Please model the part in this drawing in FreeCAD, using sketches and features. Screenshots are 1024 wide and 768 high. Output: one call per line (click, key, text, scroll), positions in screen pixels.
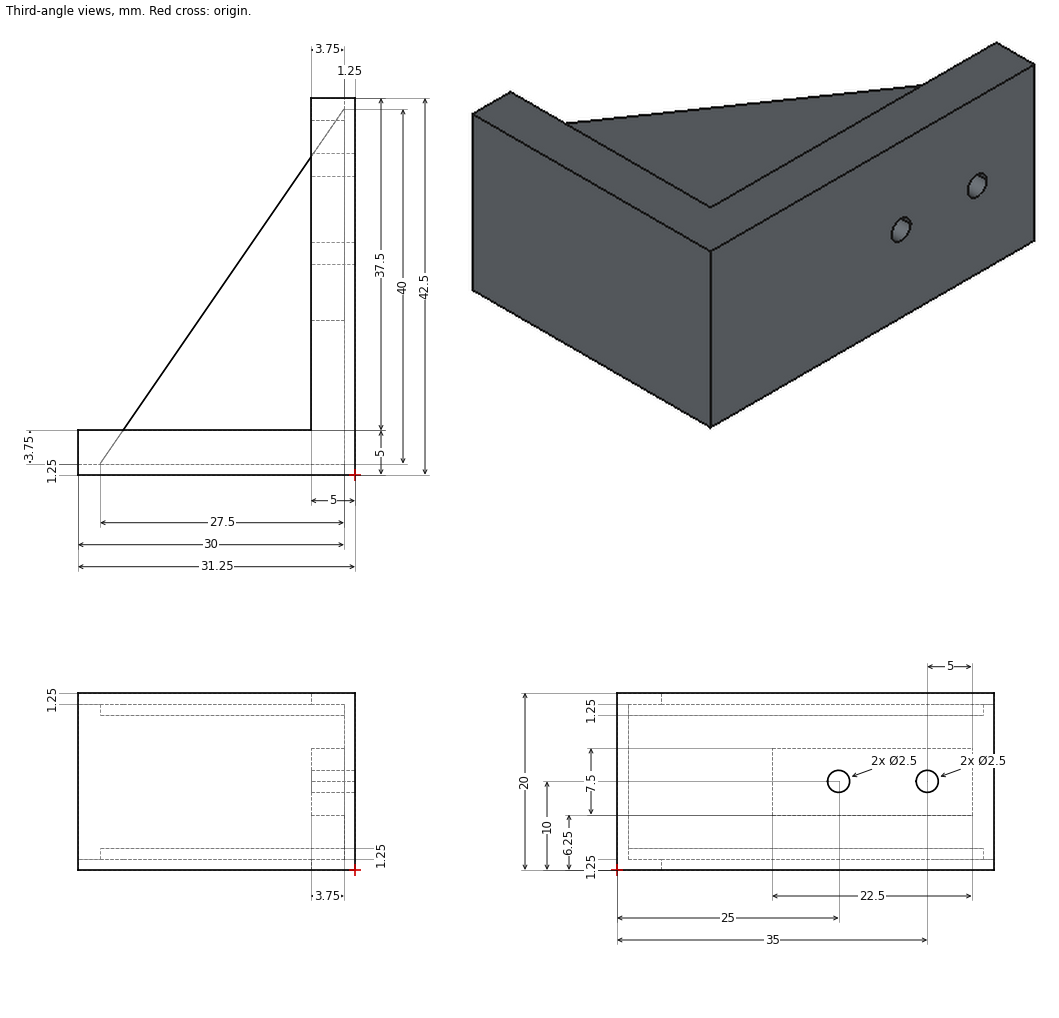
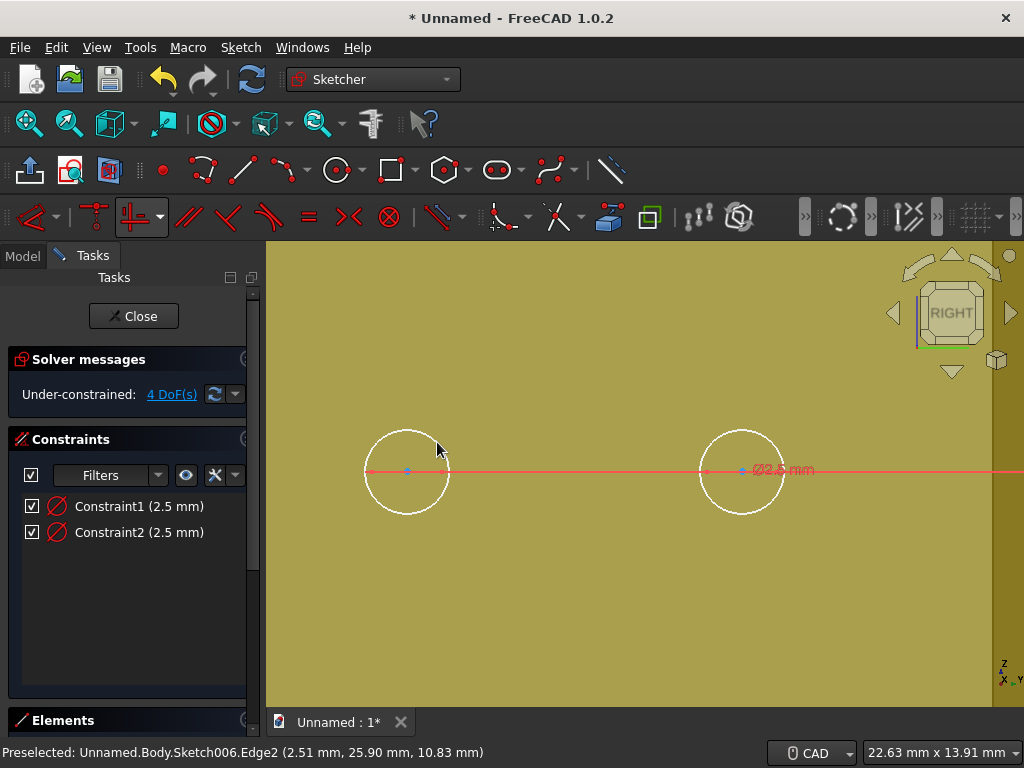
click(742, 472)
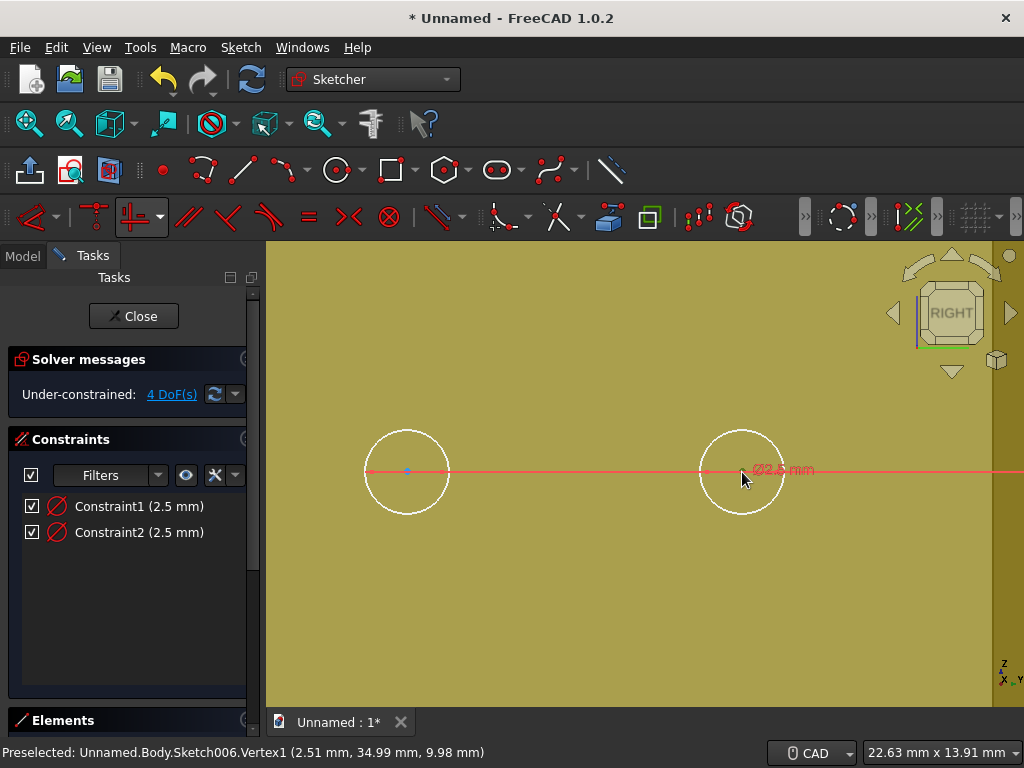
click(407, 472)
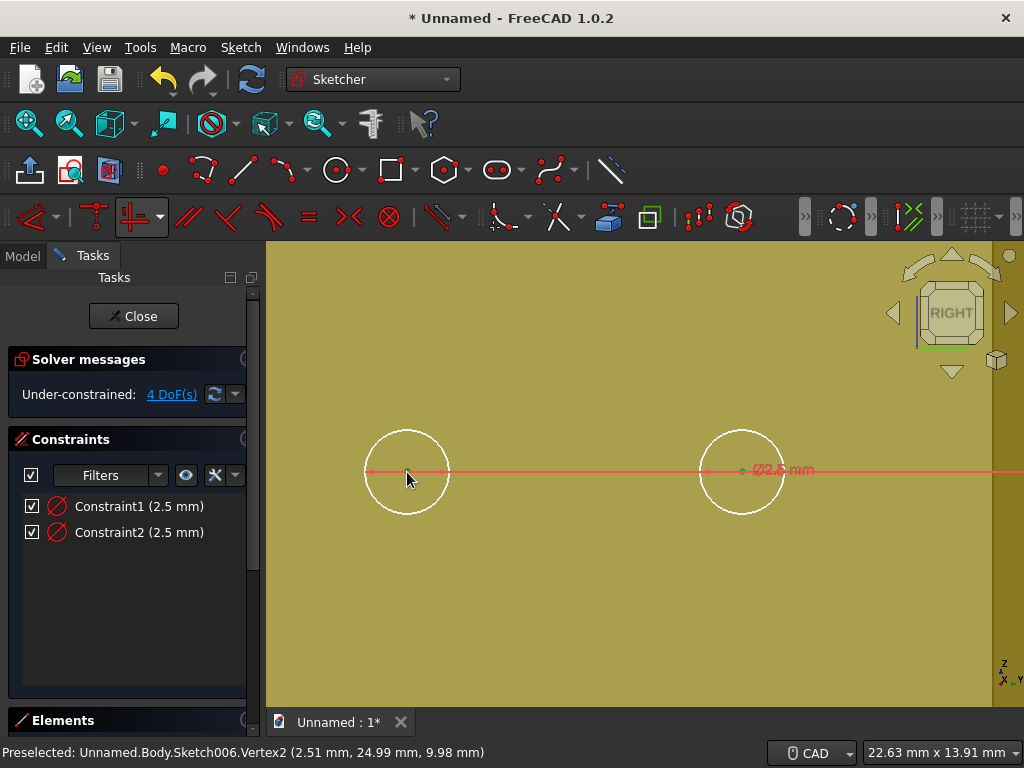
click(162, 218)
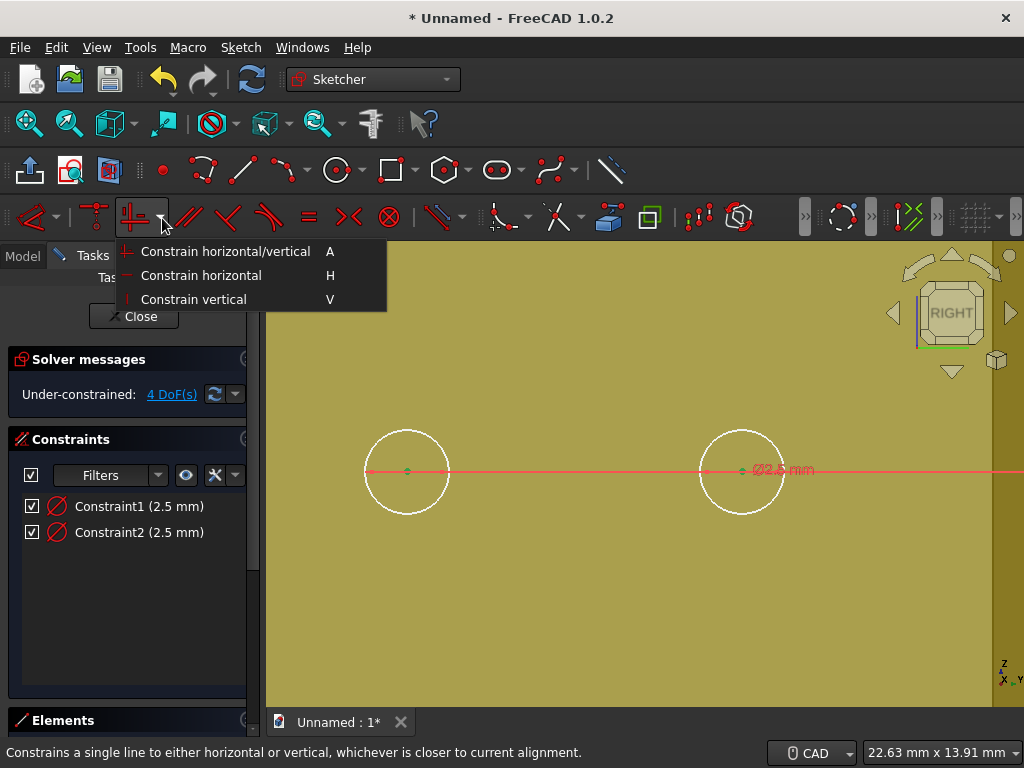
click(251, 275)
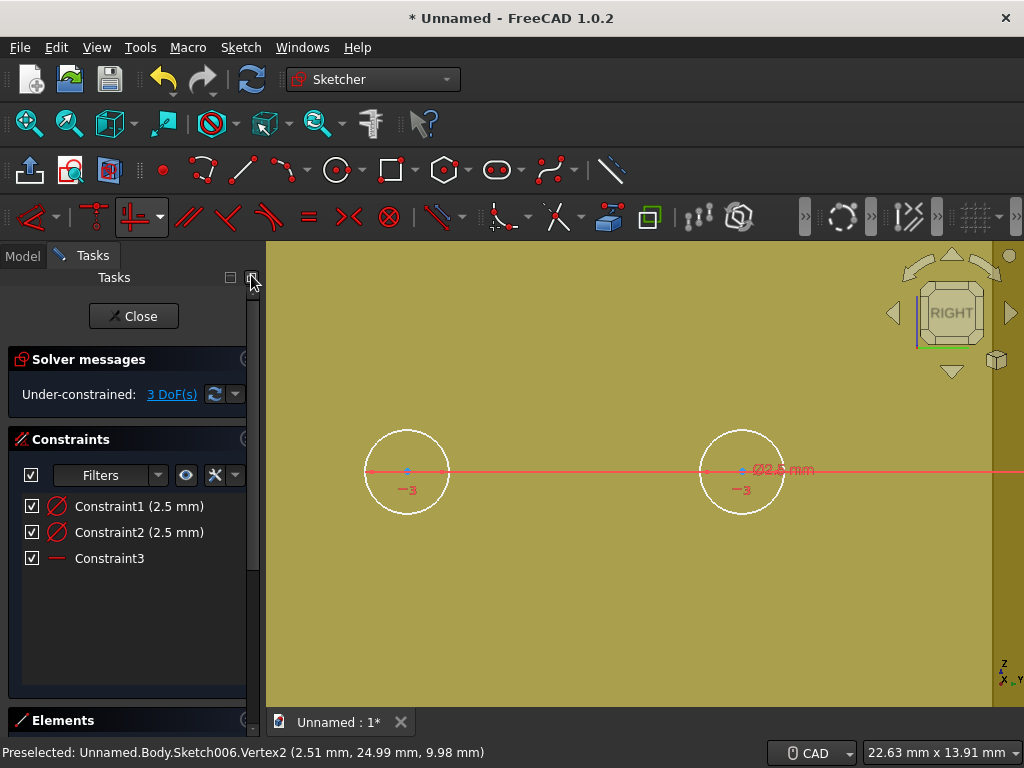
click(32, 218)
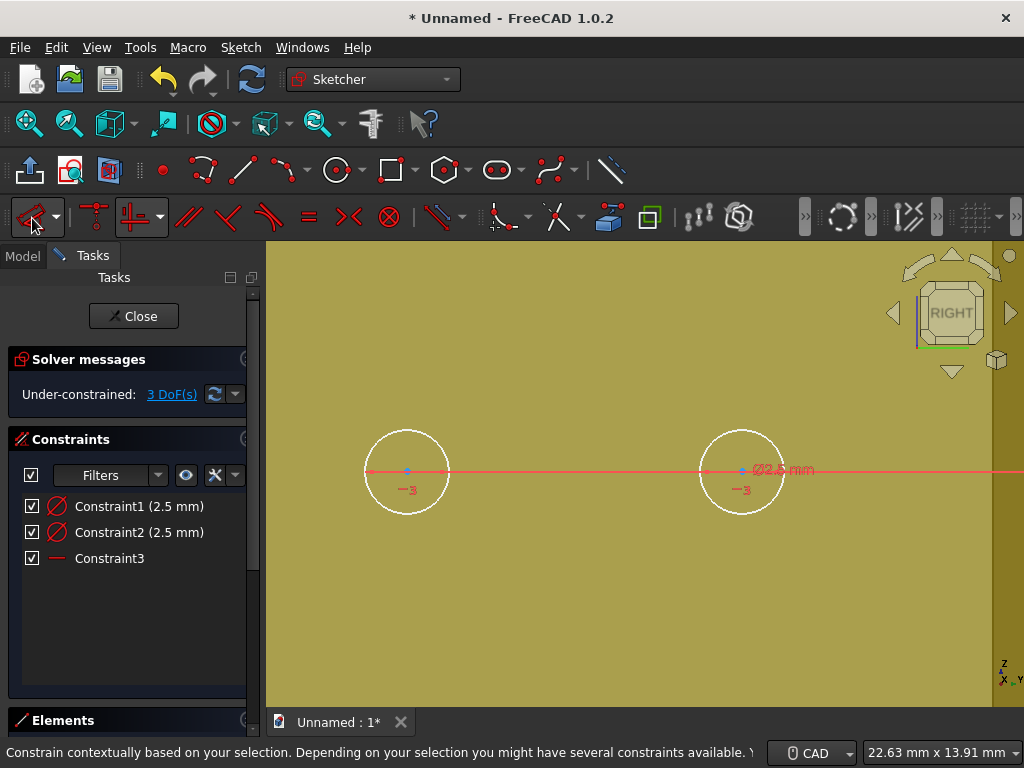
click(742, 472)
click(518, 438)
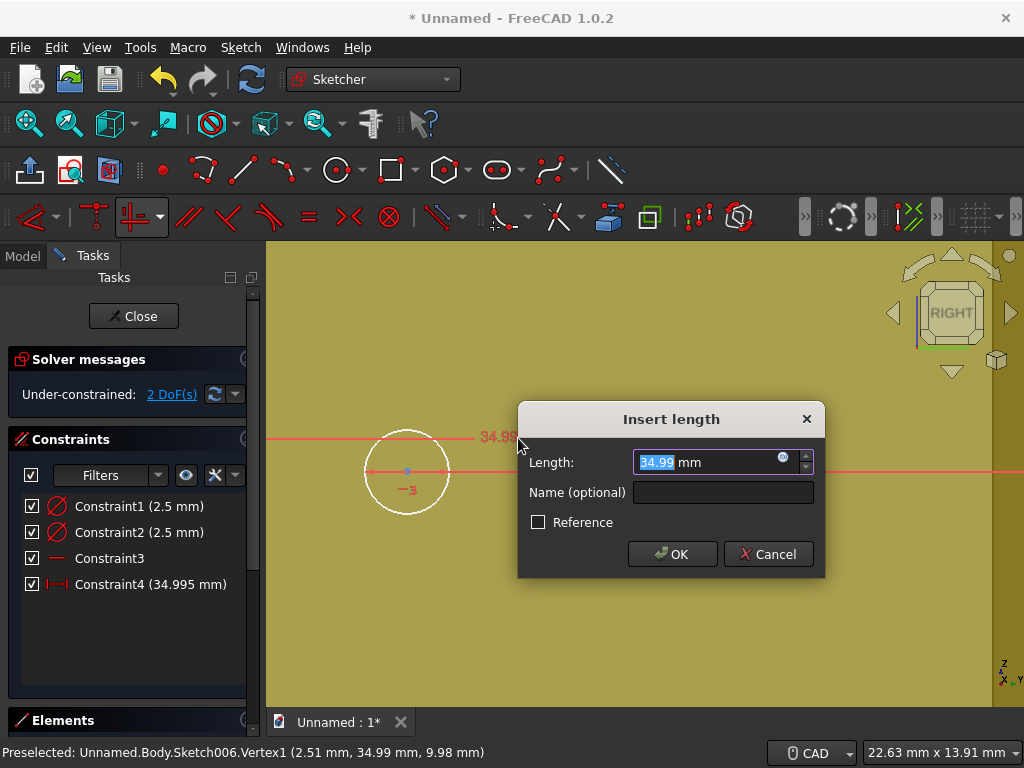
text(35)
key(Return)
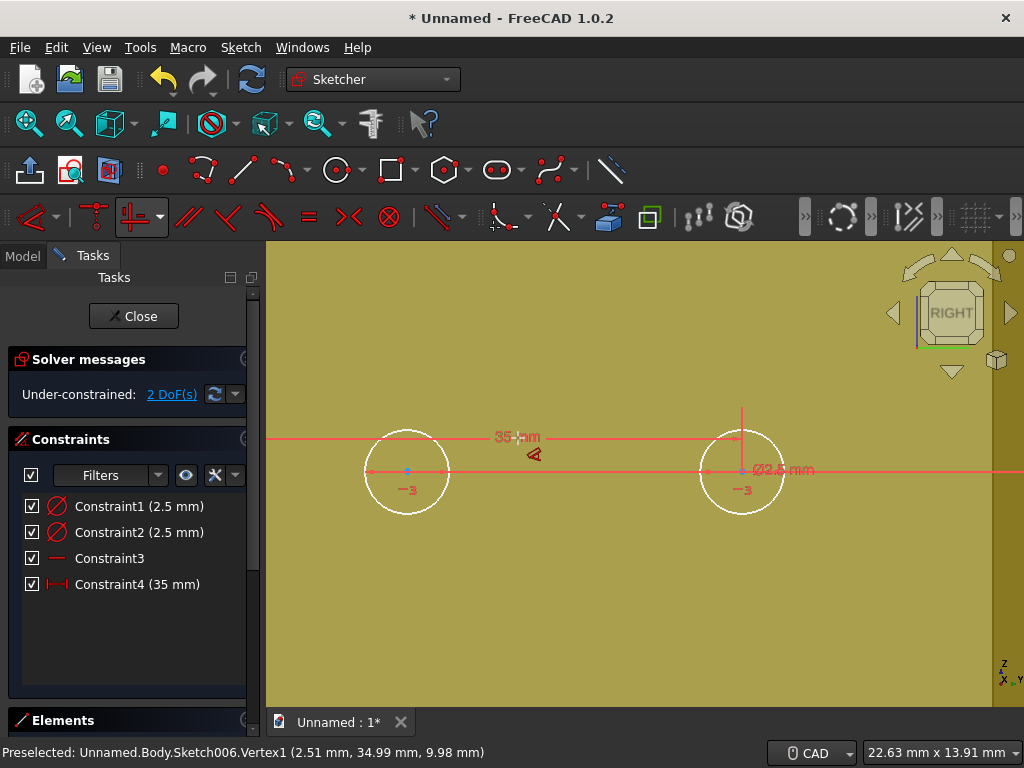
click(742, 472)
click(776, 576)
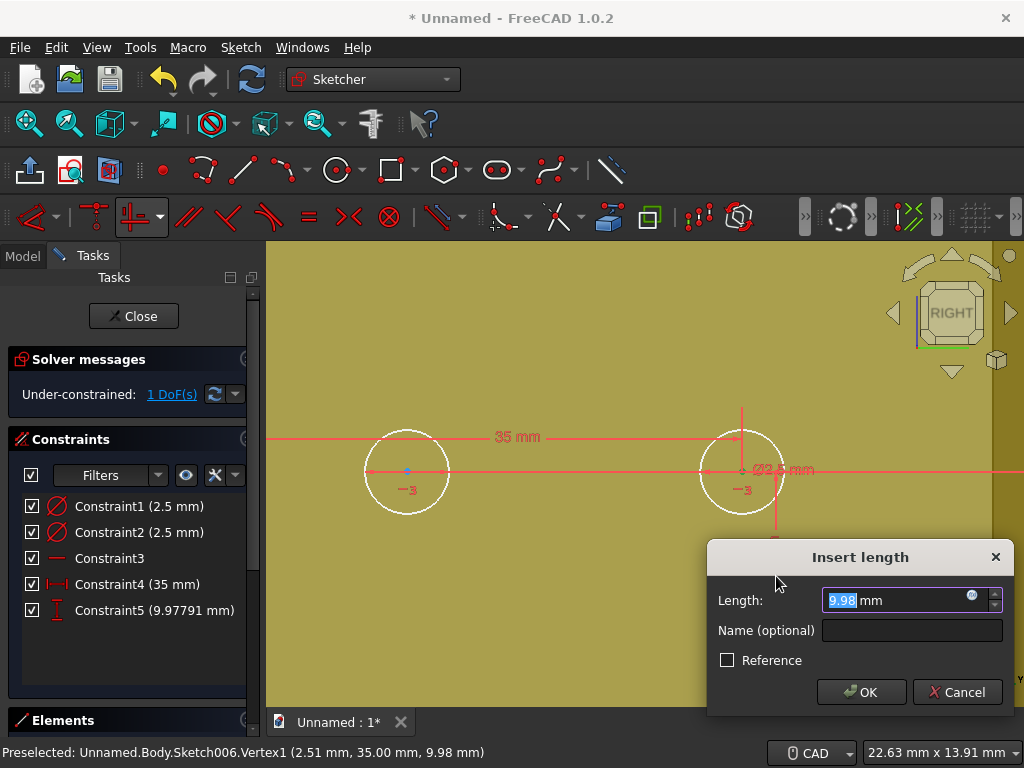
text(10)
key(Return)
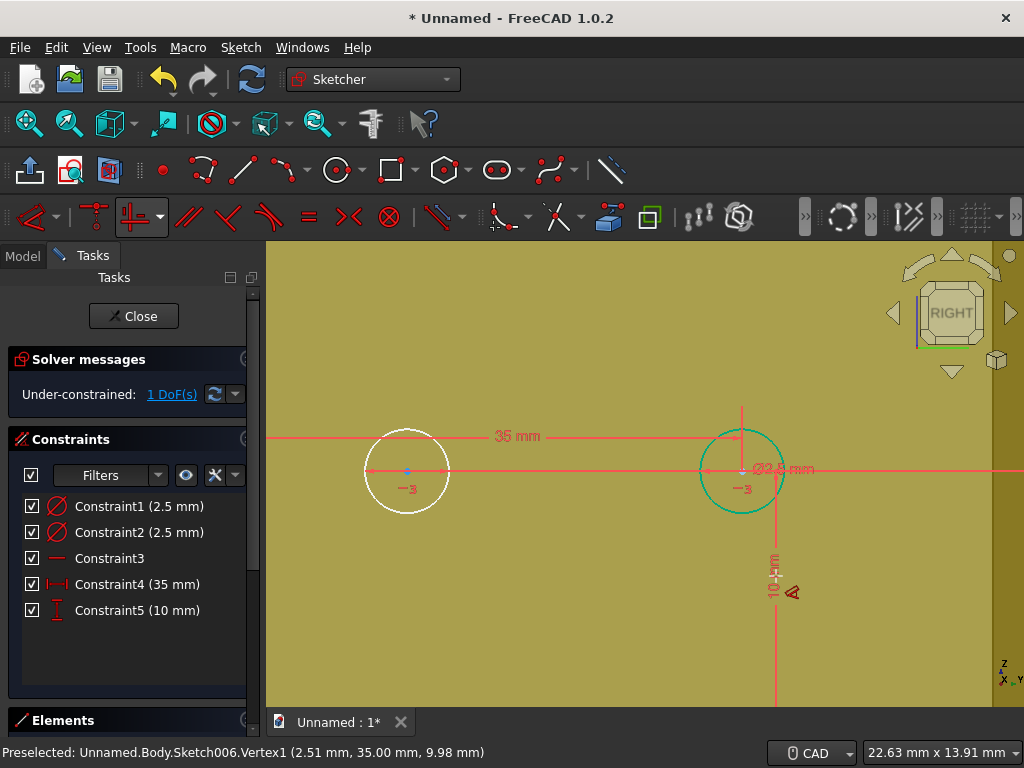
click(407, 471)
click(351, 437)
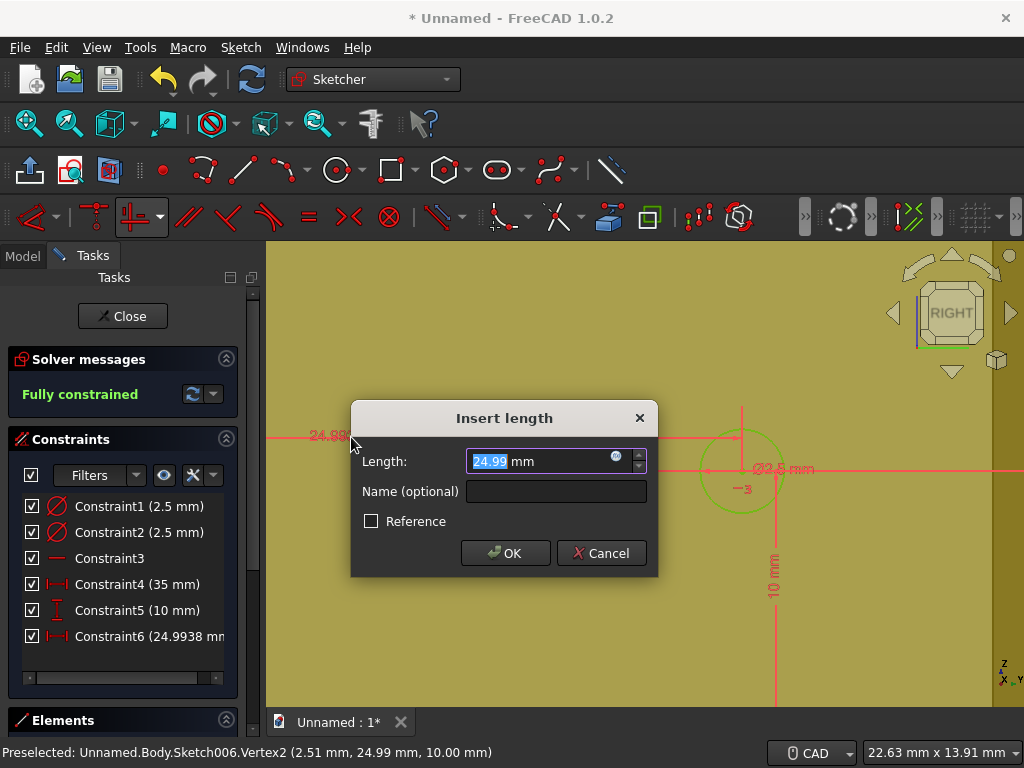
text(25)
key(Return)
key(Escape)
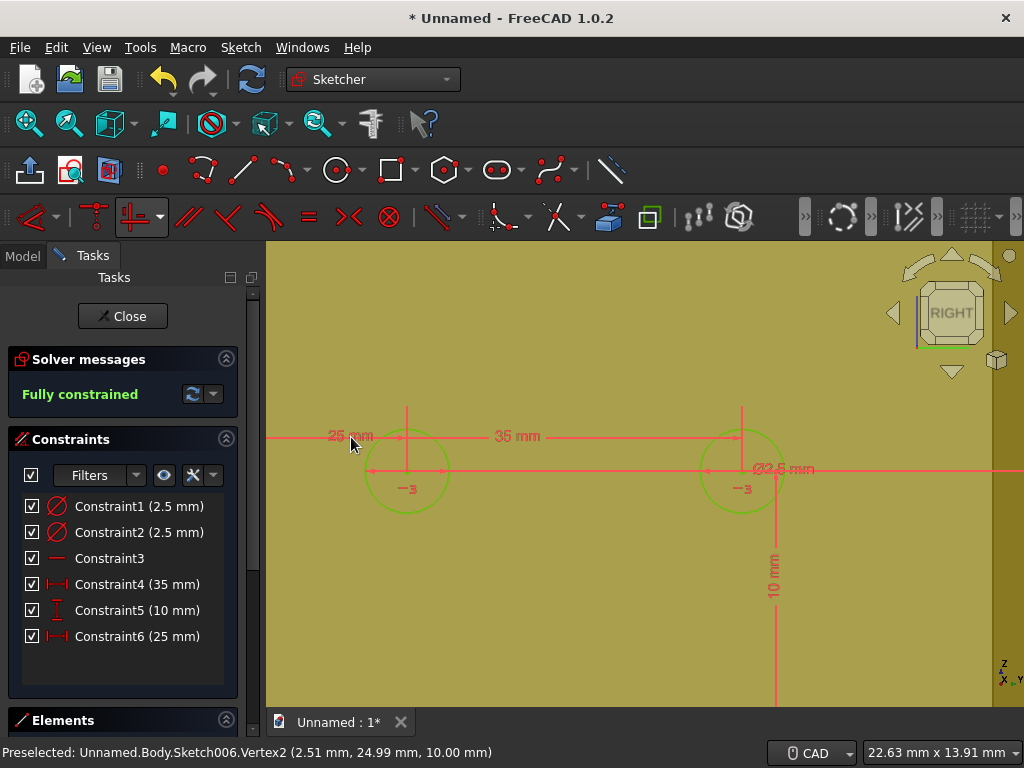
click(123, 316)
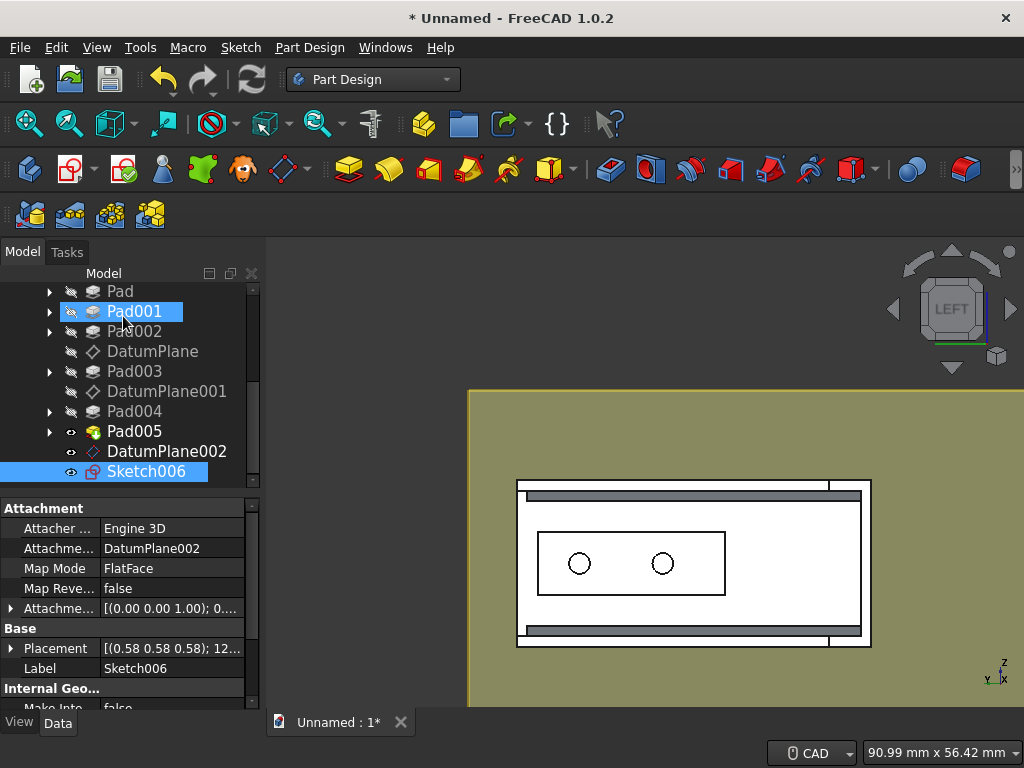
click(612, 170)